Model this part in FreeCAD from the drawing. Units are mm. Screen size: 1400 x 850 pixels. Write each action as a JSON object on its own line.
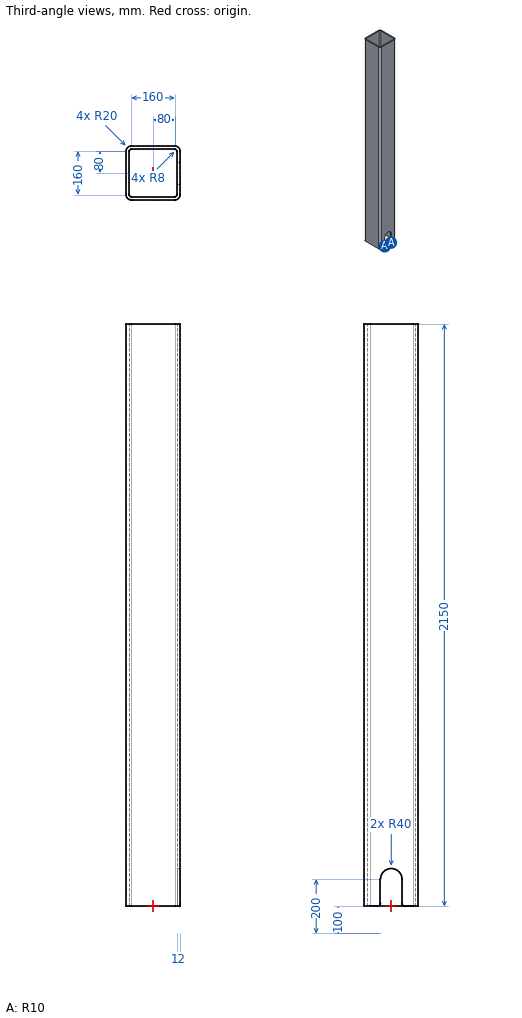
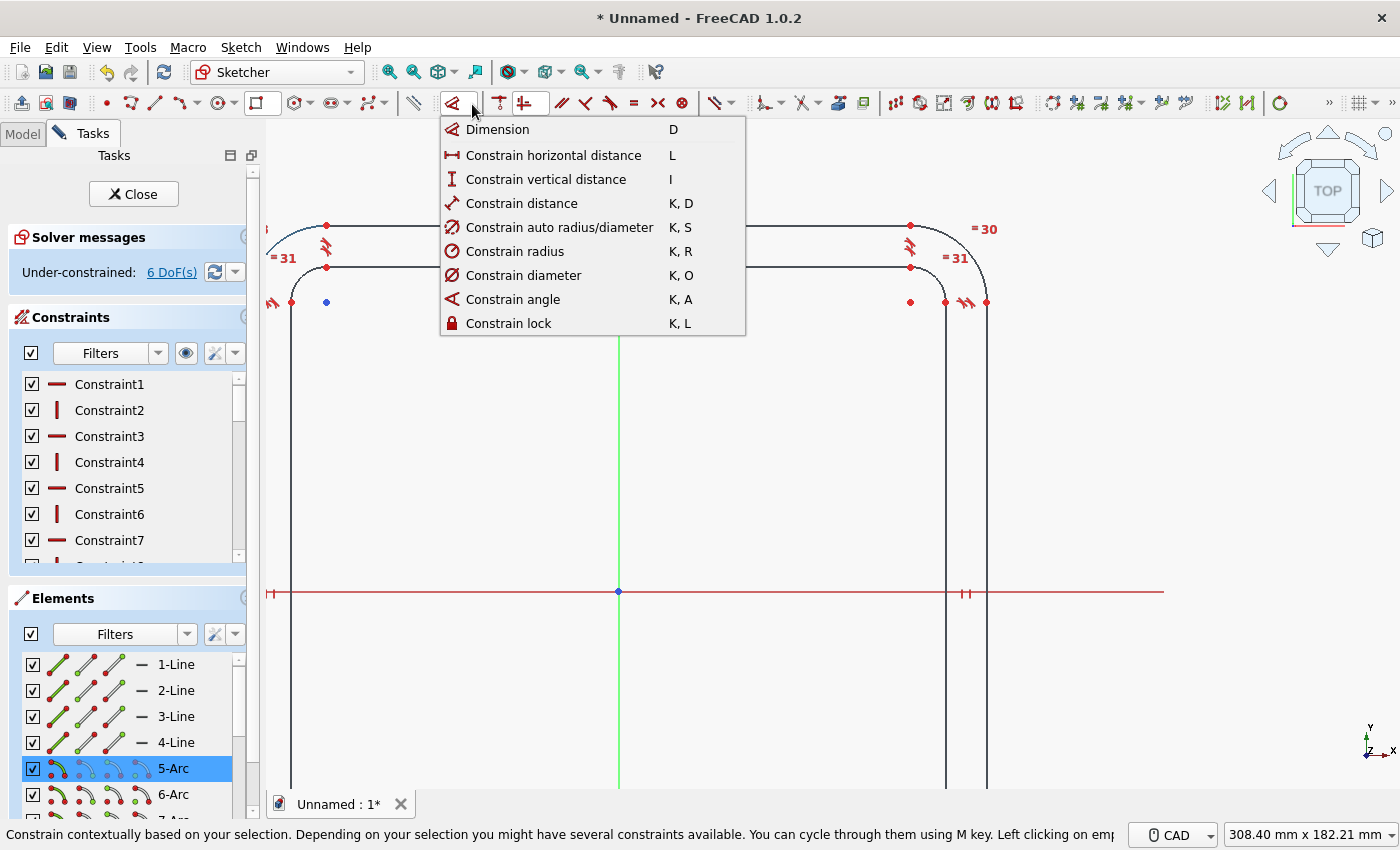
{"action": "left_click", "coordinate": [593, 251]}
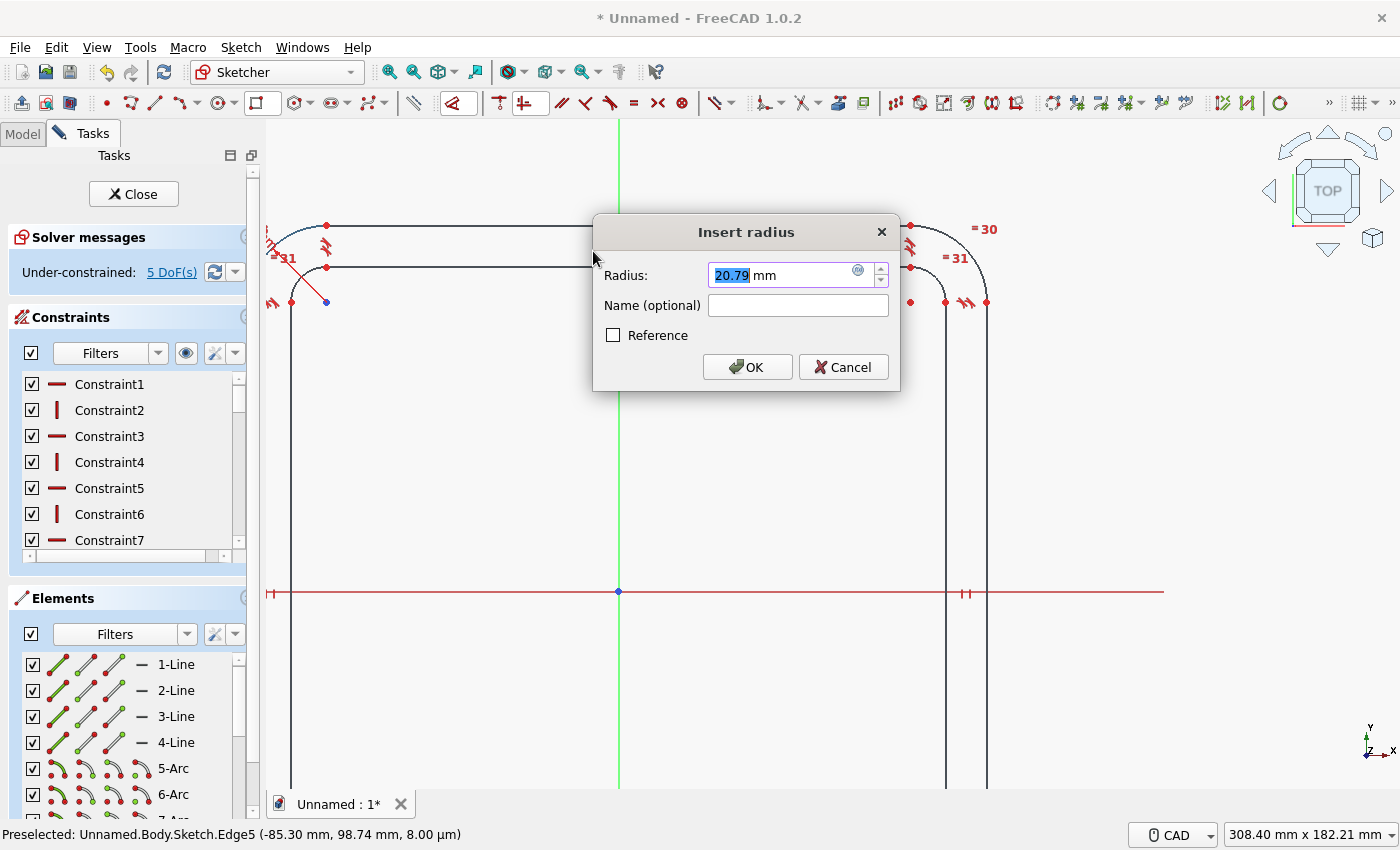
{"action": "type", "text": "20"}
{"action": "key", "text": "Return"}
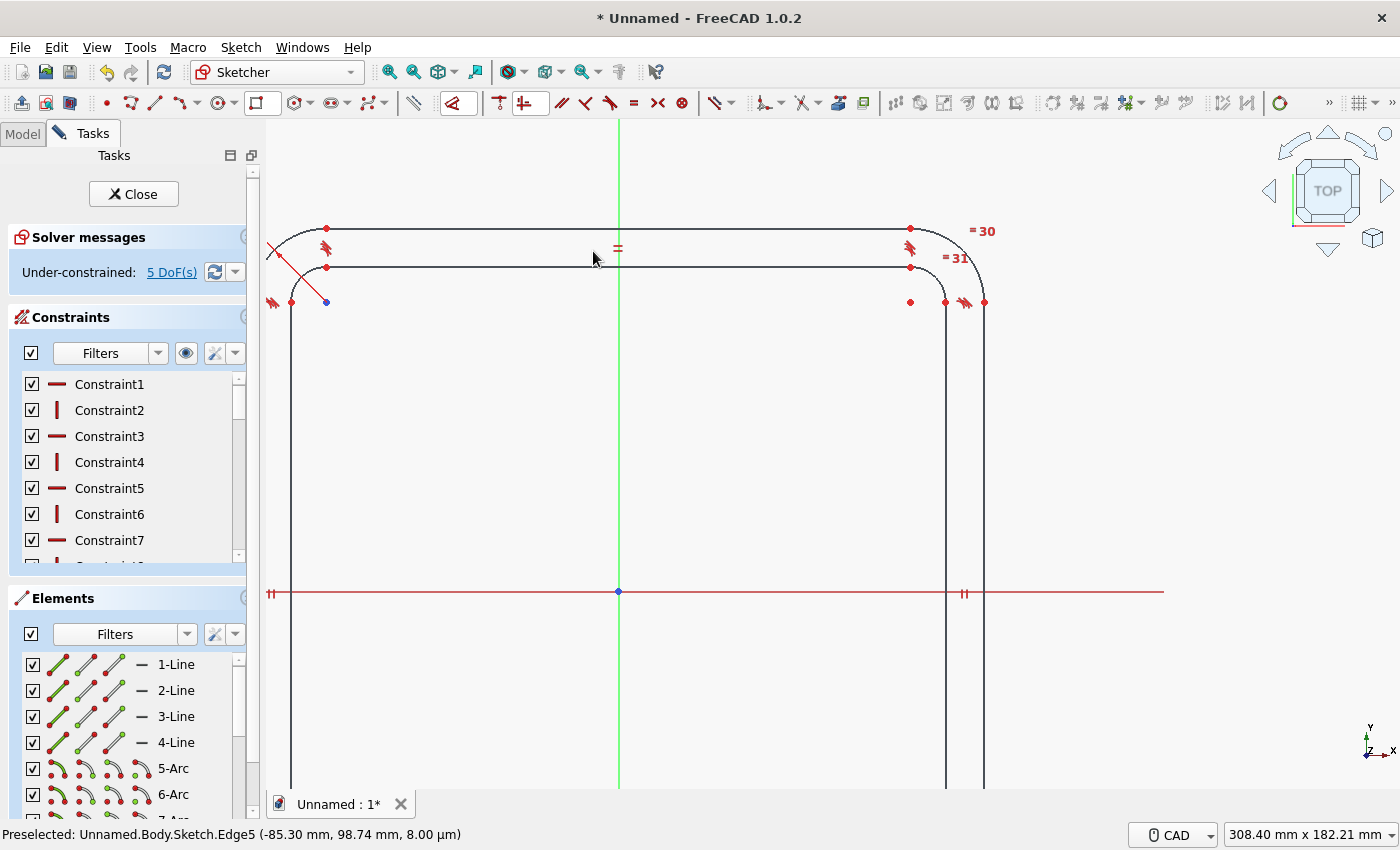
{"action": "scroll", "coordinate": [942, 286], "scroll_direction": "up", "scroll_amount": 2}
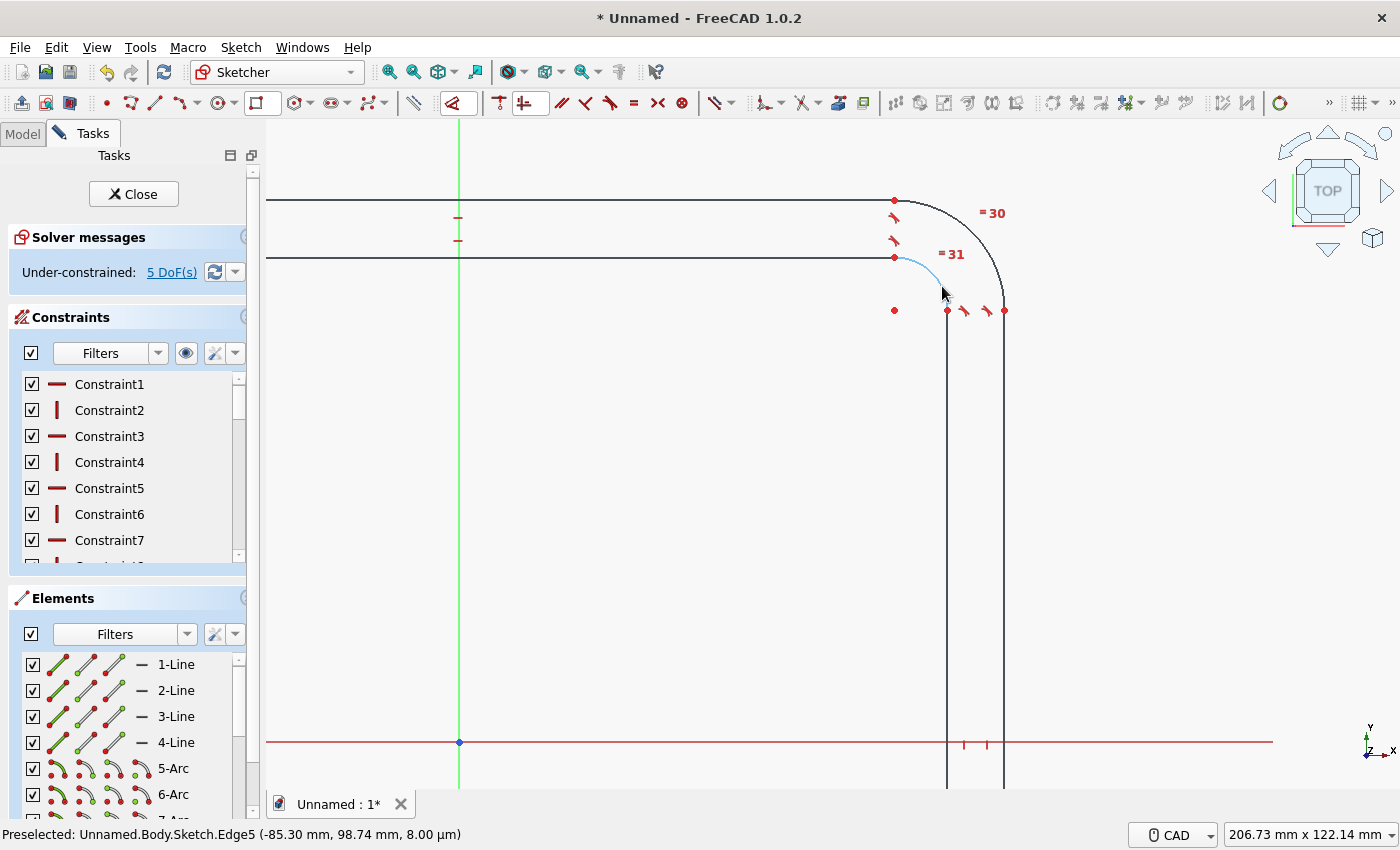
{"action": "left_click", "coordinate": [942, 286]}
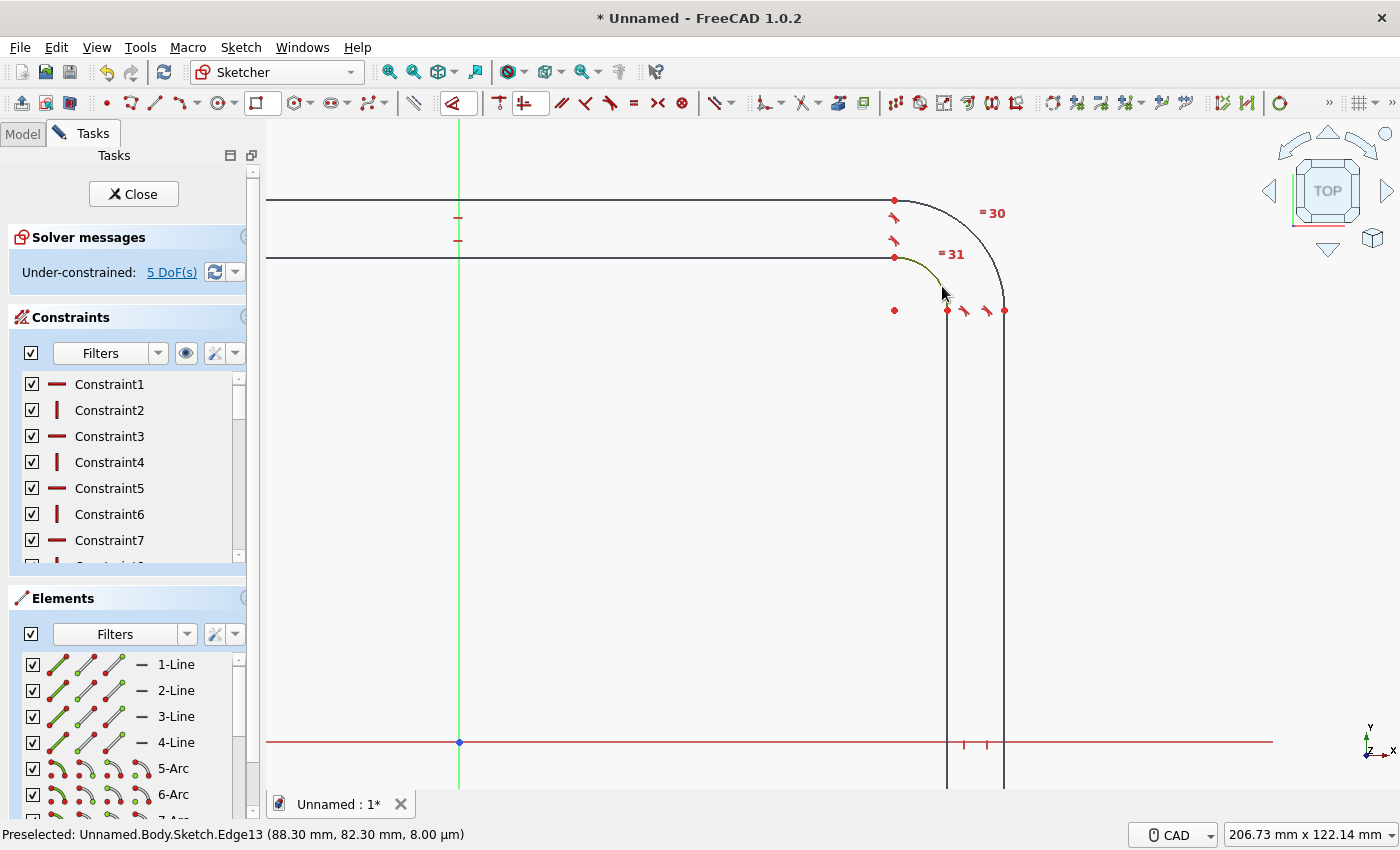
{"action": "left_click", "coordinate": [472, 104]}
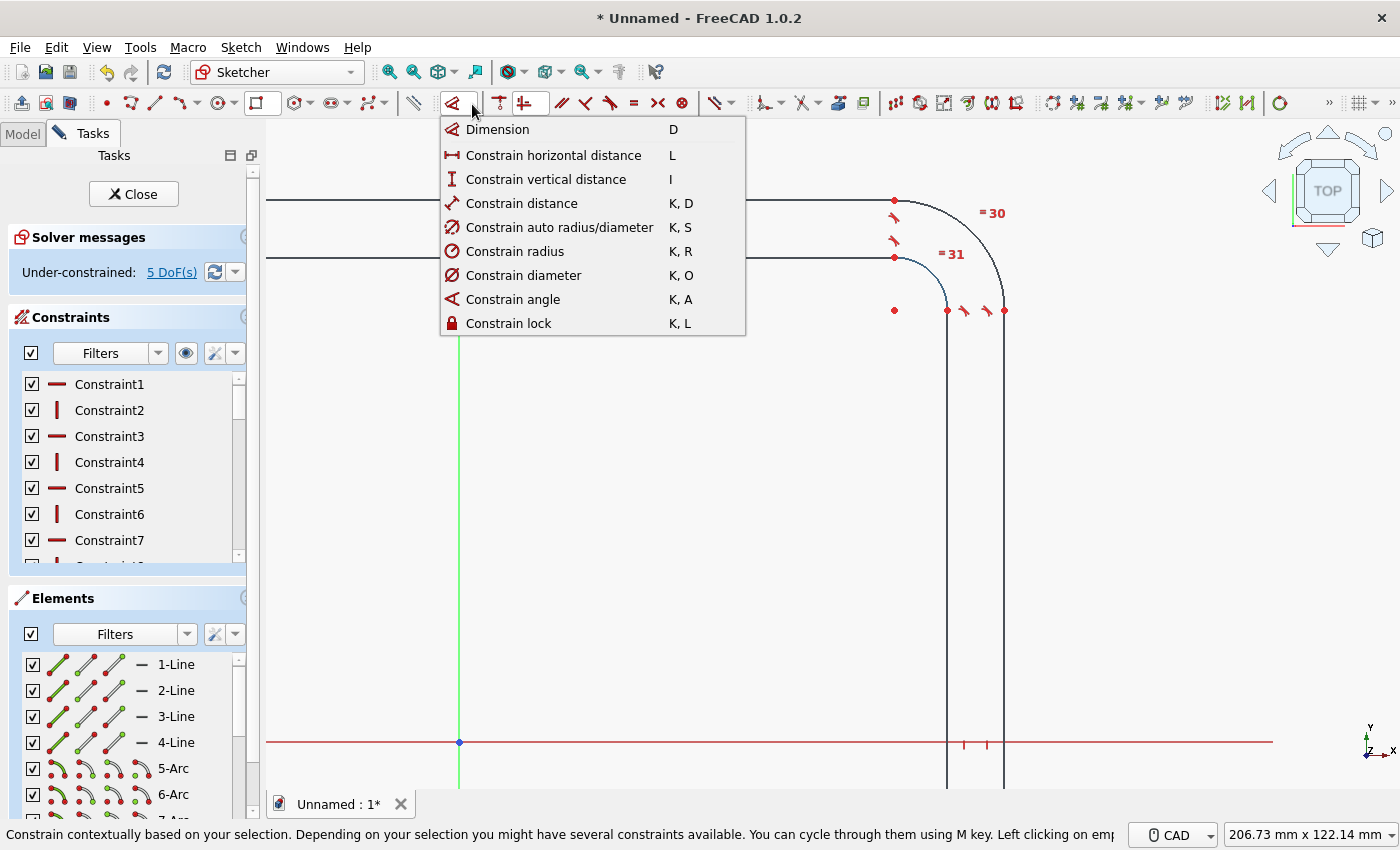
{"action": "left_click", "coordinate": [593, 251]}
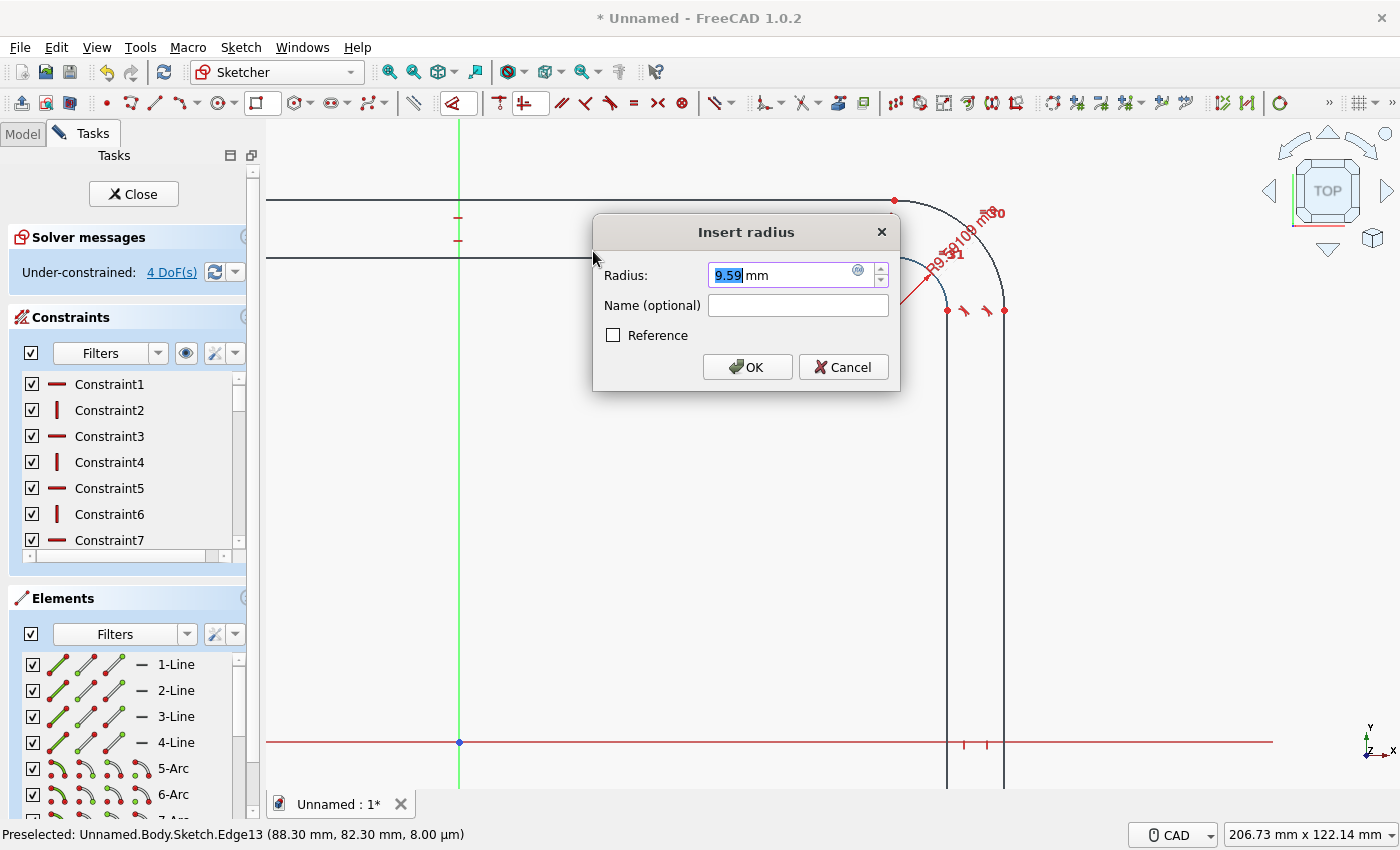
{"action": "type", "text": "8"}
{"action": "key", "text": "Return"}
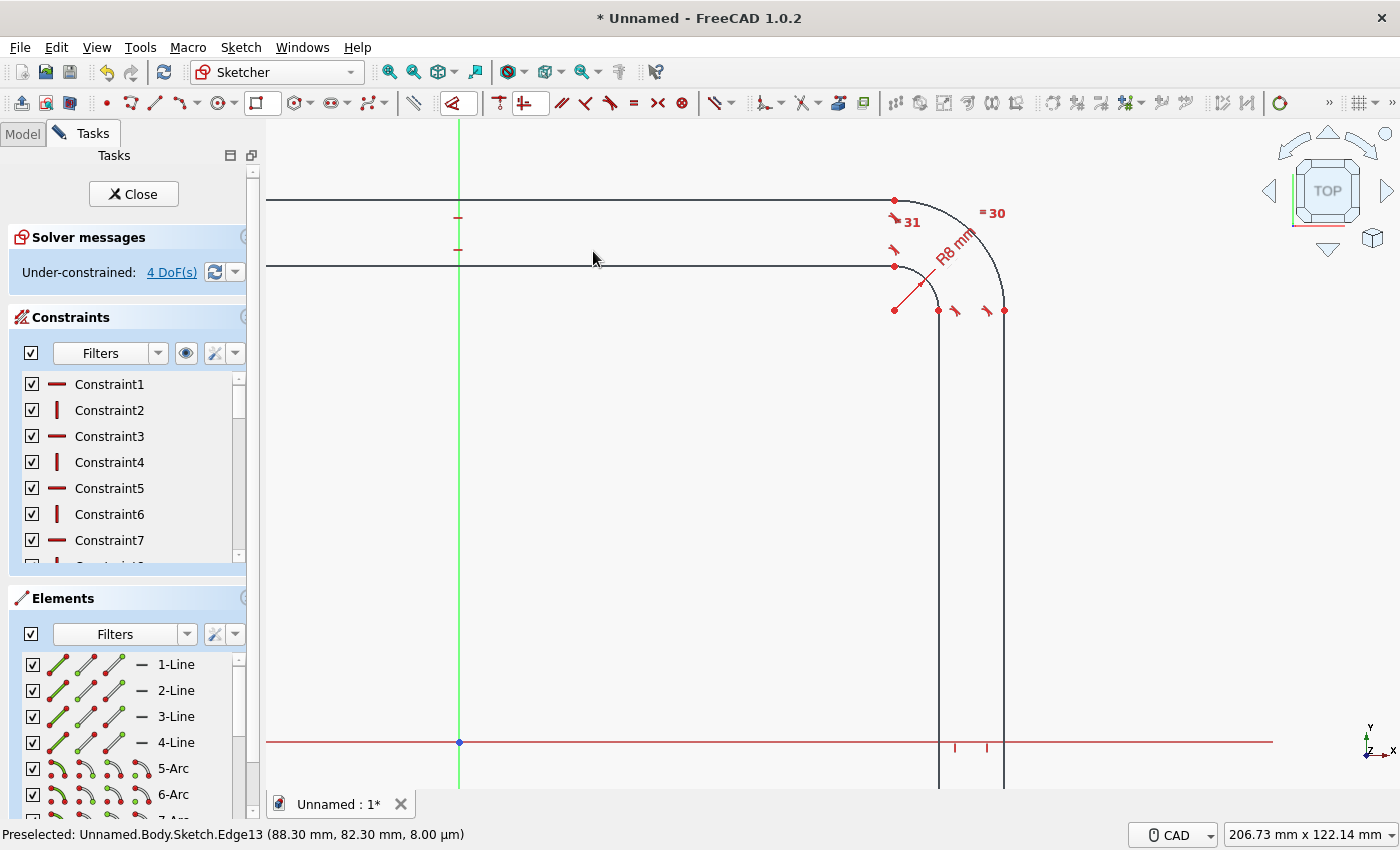
{"action": "left_click", "coordinate": [633, 200]}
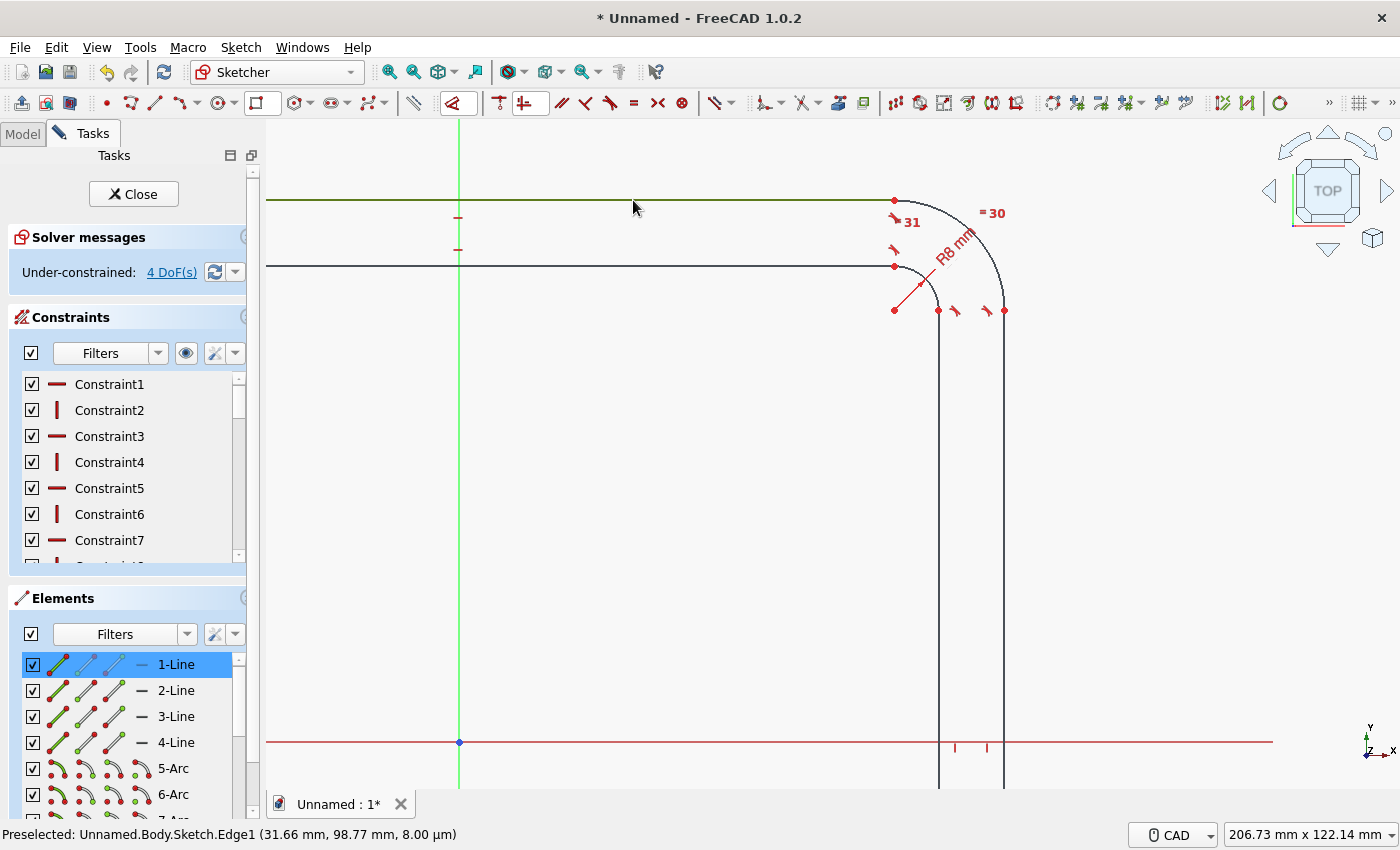
{"action": "key", "text": "l"}